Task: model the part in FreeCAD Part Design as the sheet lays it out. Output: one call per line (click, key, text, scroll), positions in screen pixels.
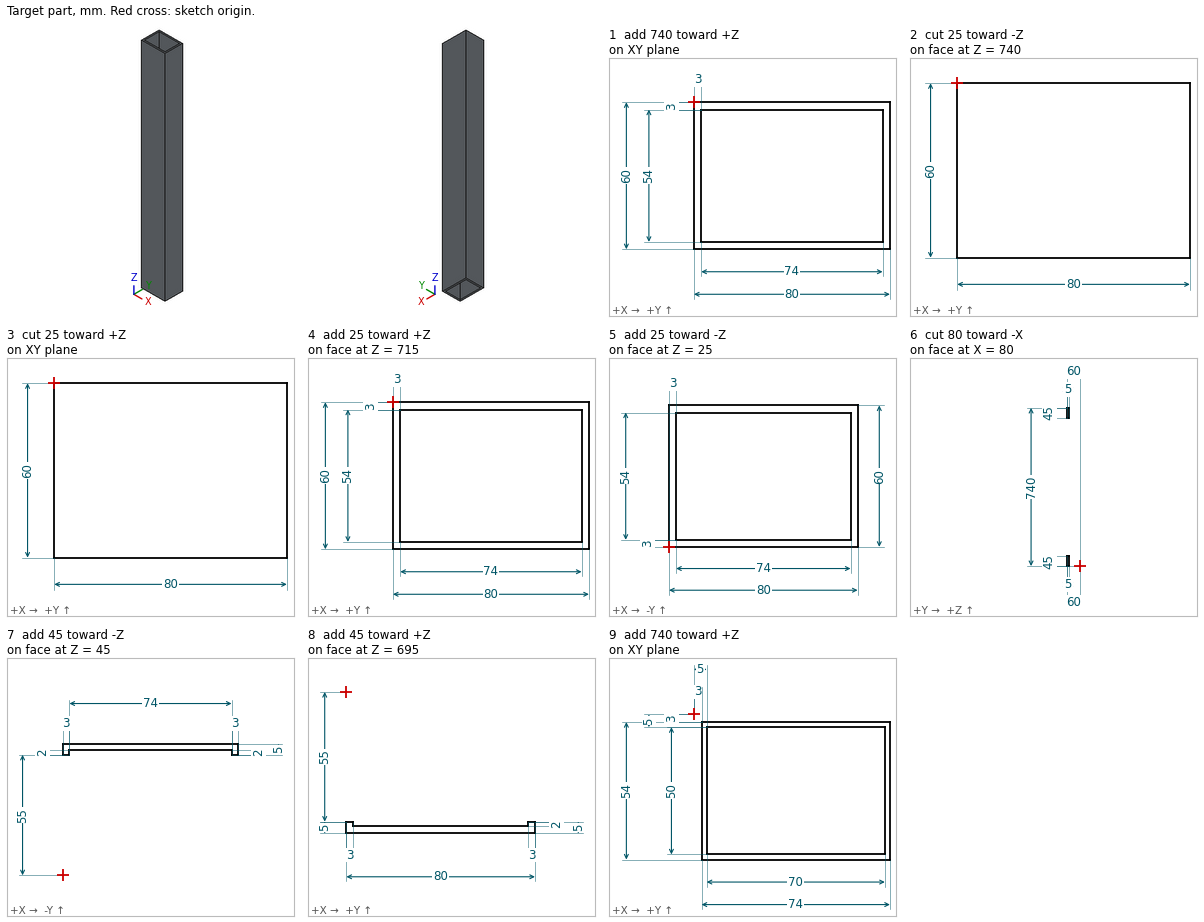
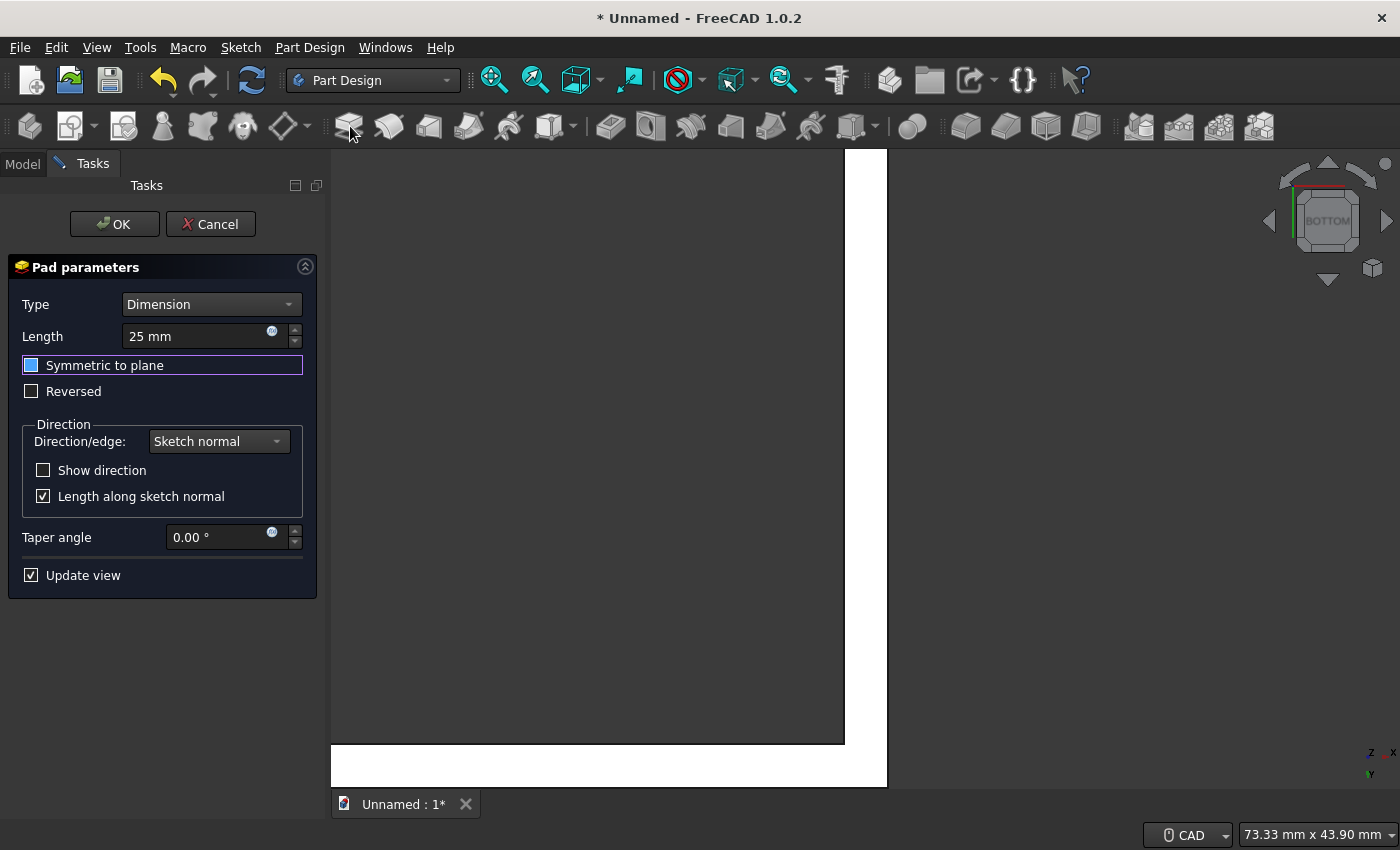
click(115, 224)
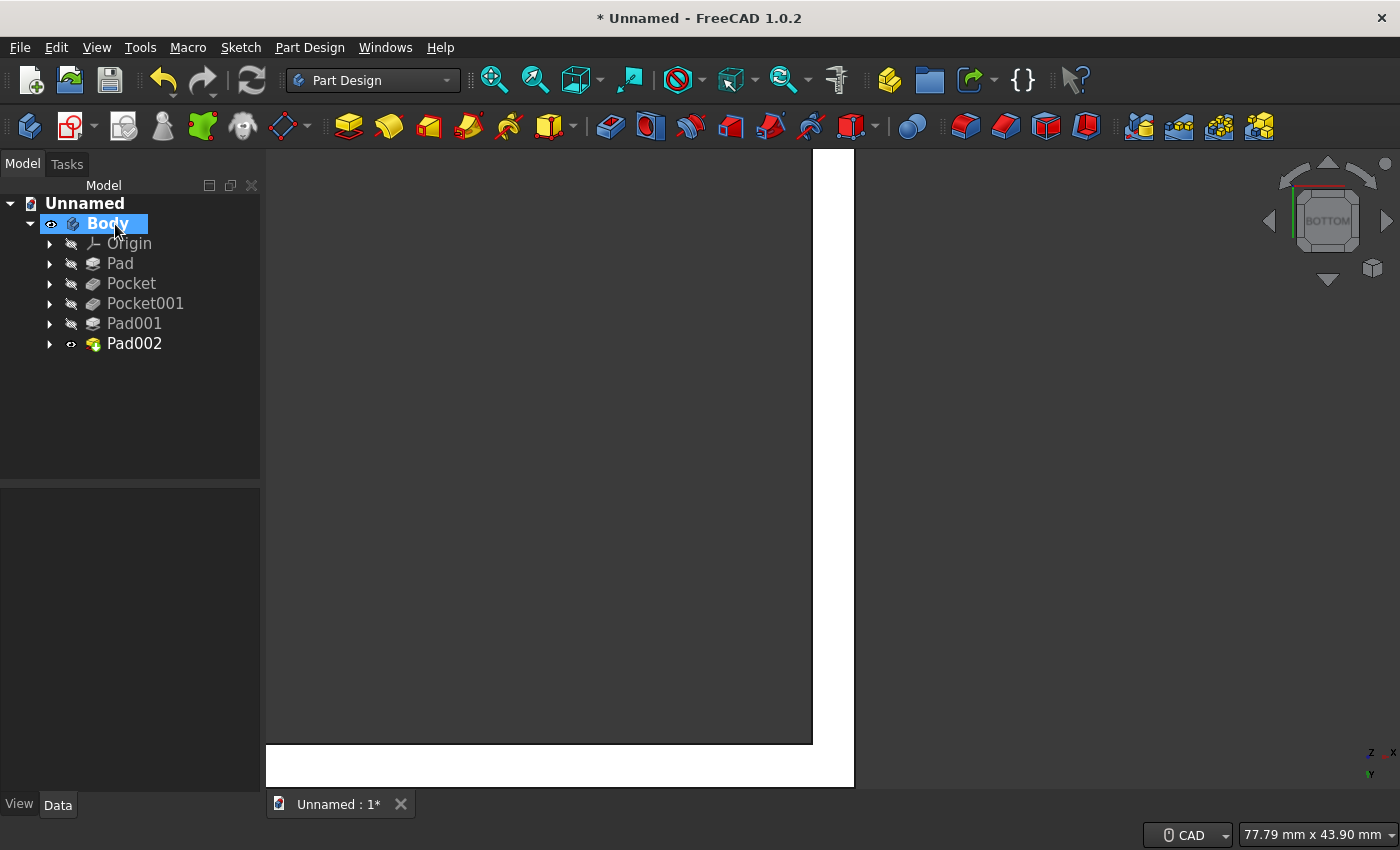
click(496, 80)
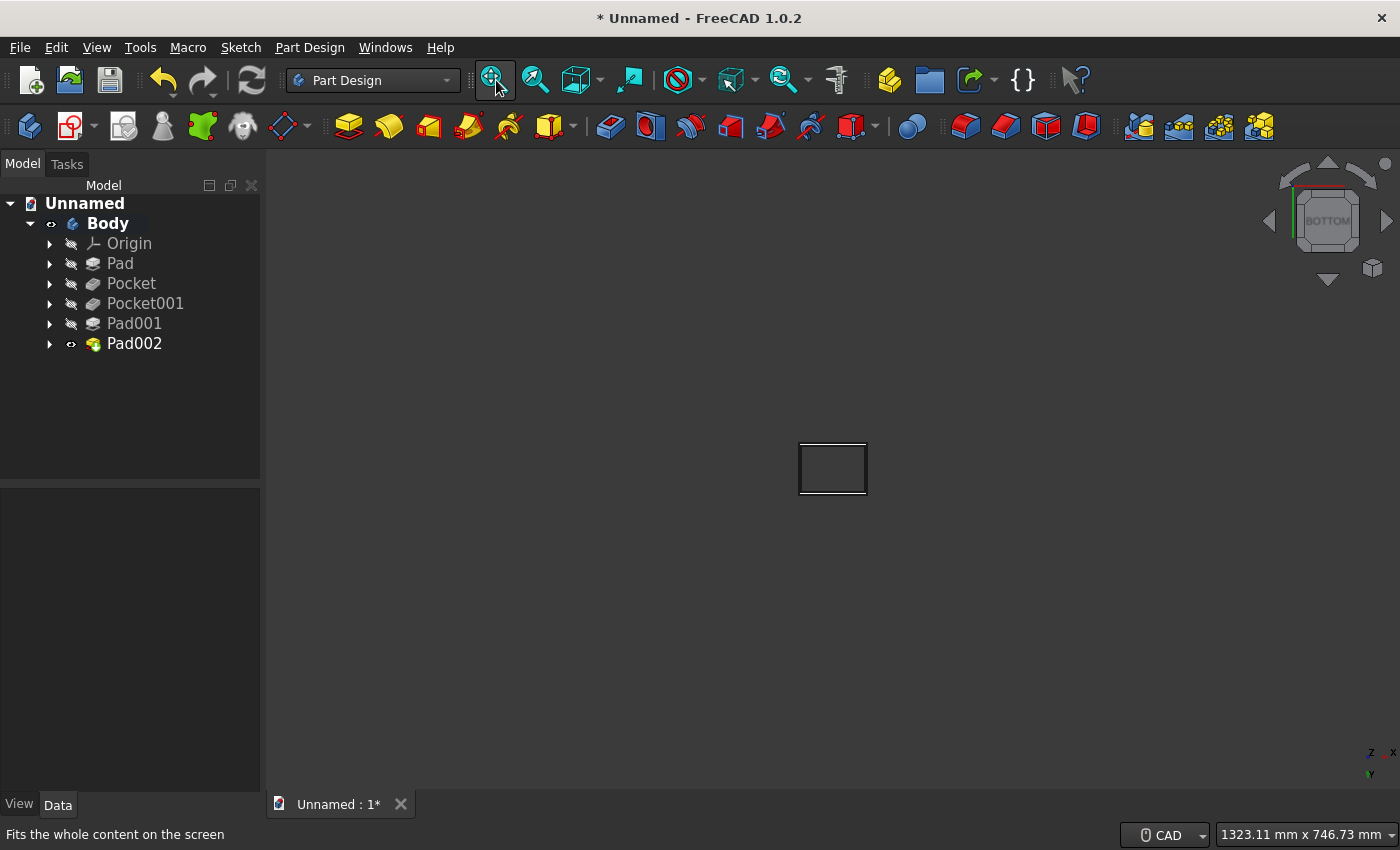
key(0)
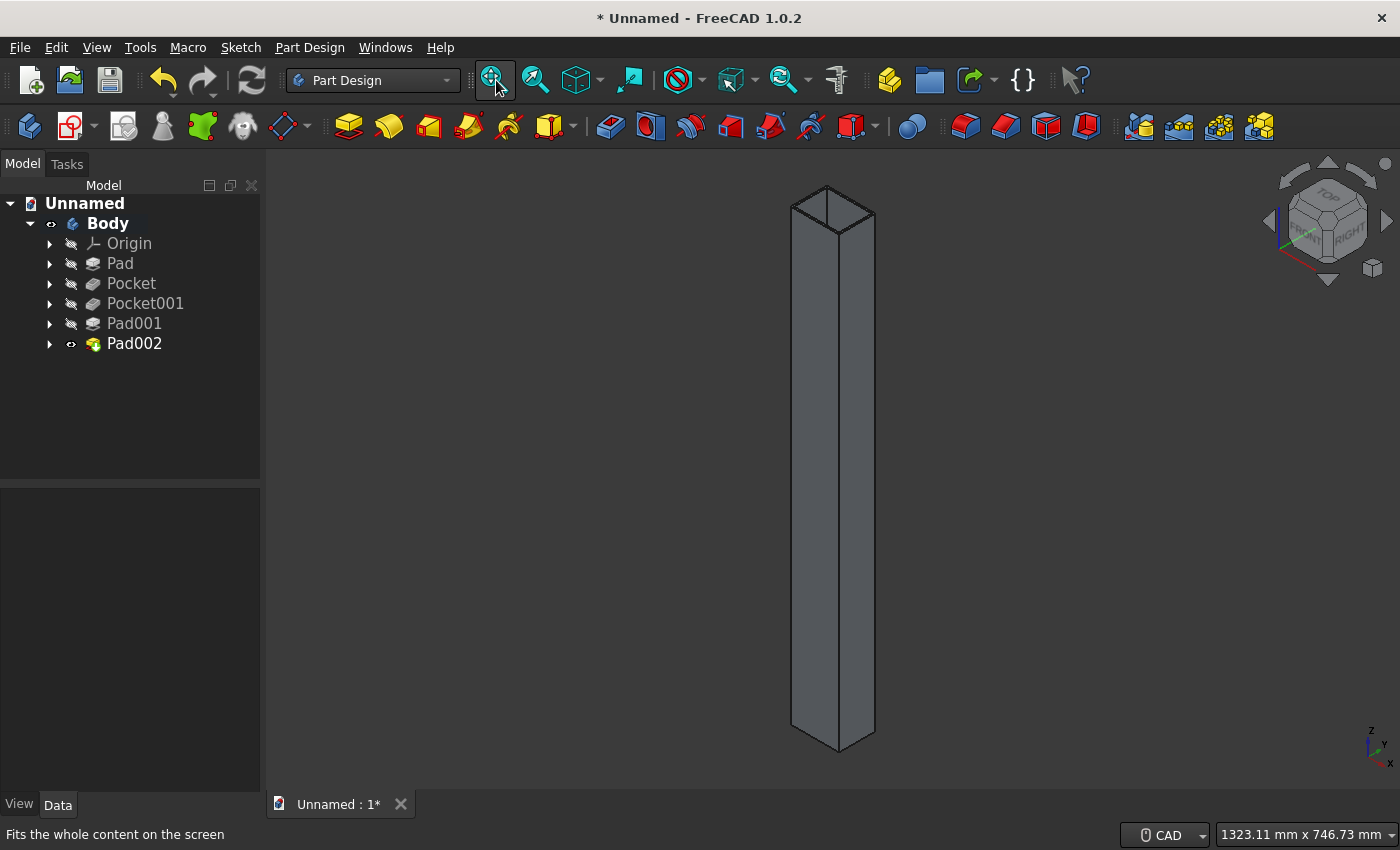
click(857, 260)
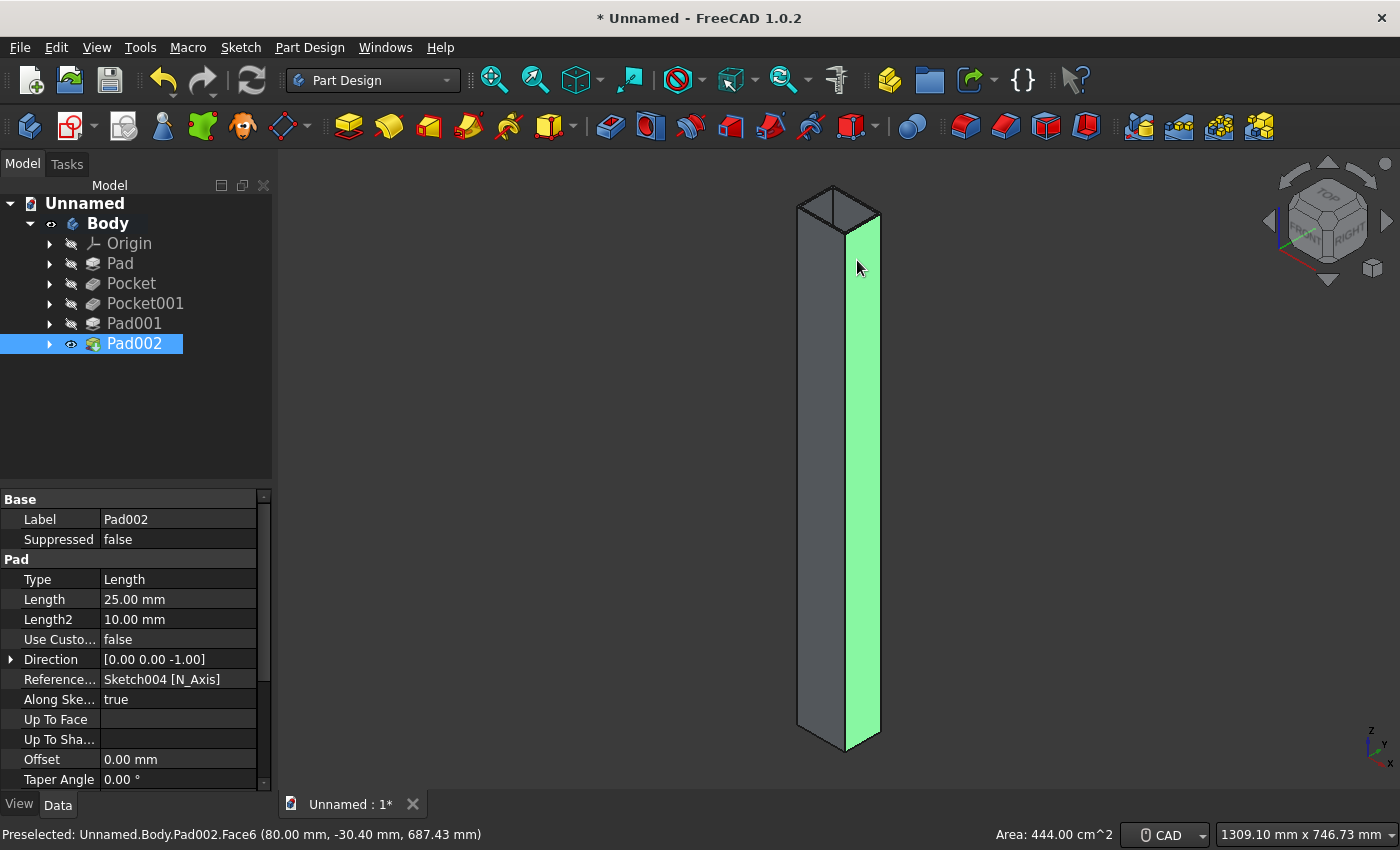
click(70, 126)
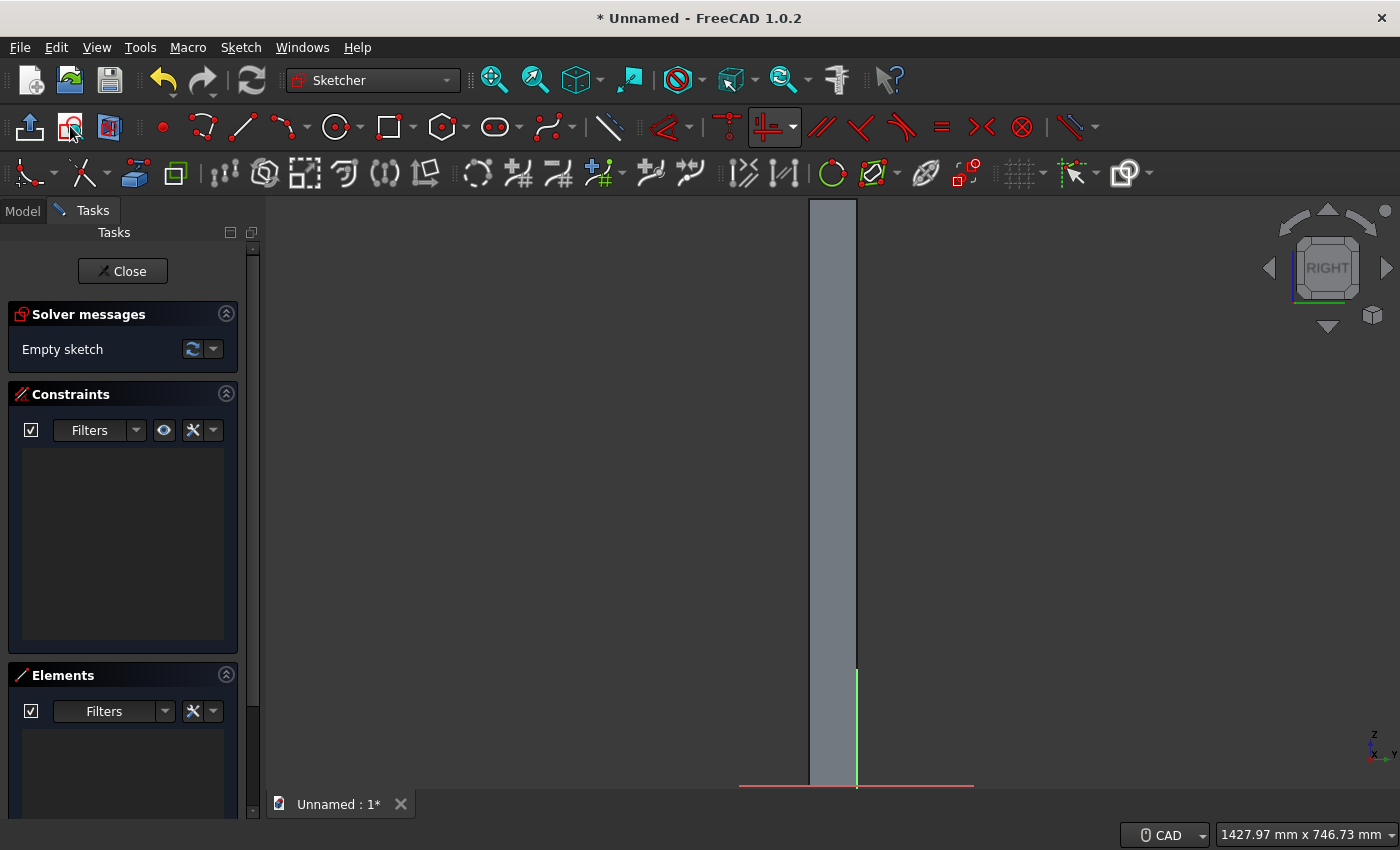
scroll(625, 493, down, 2)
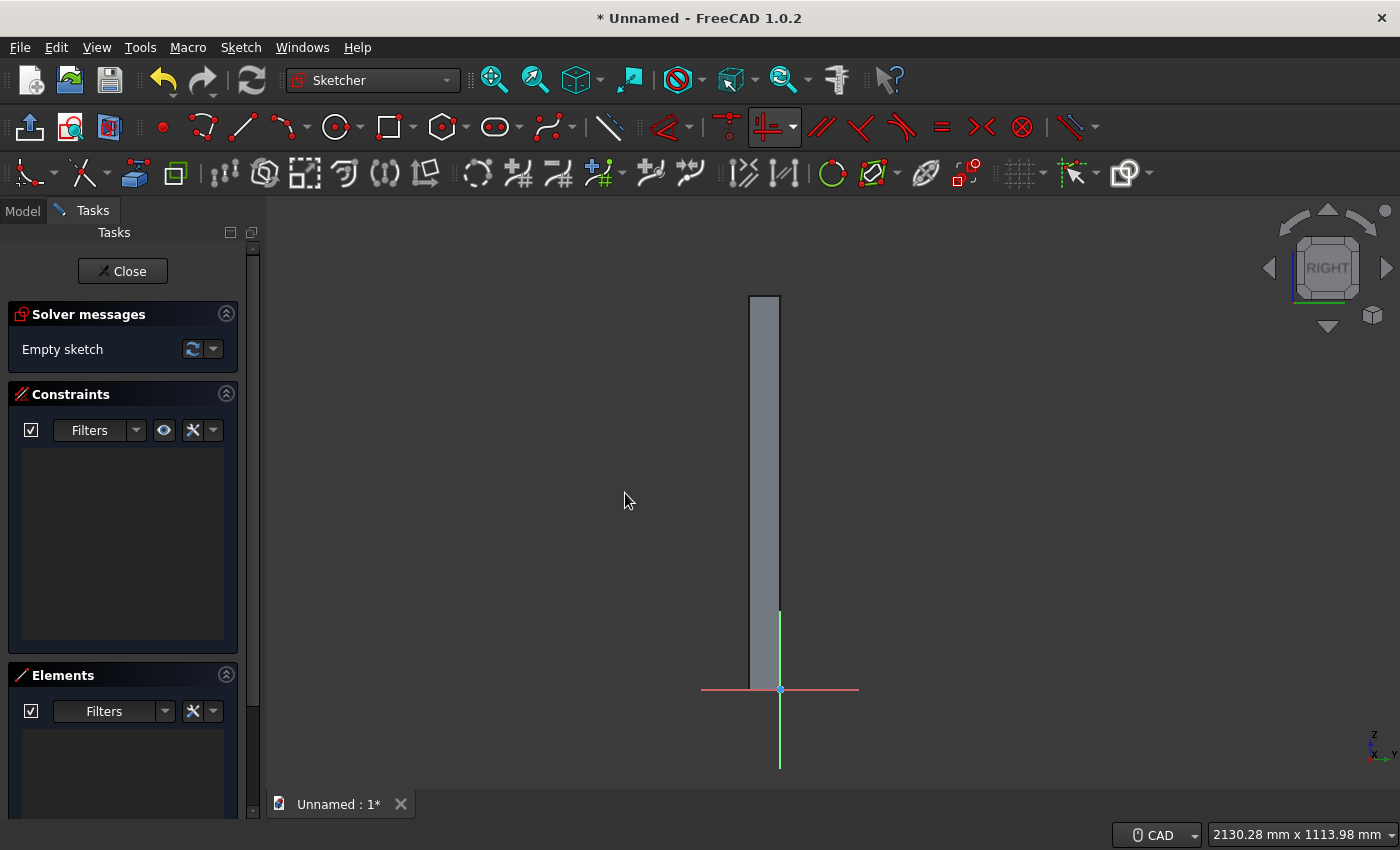
click(390, 128)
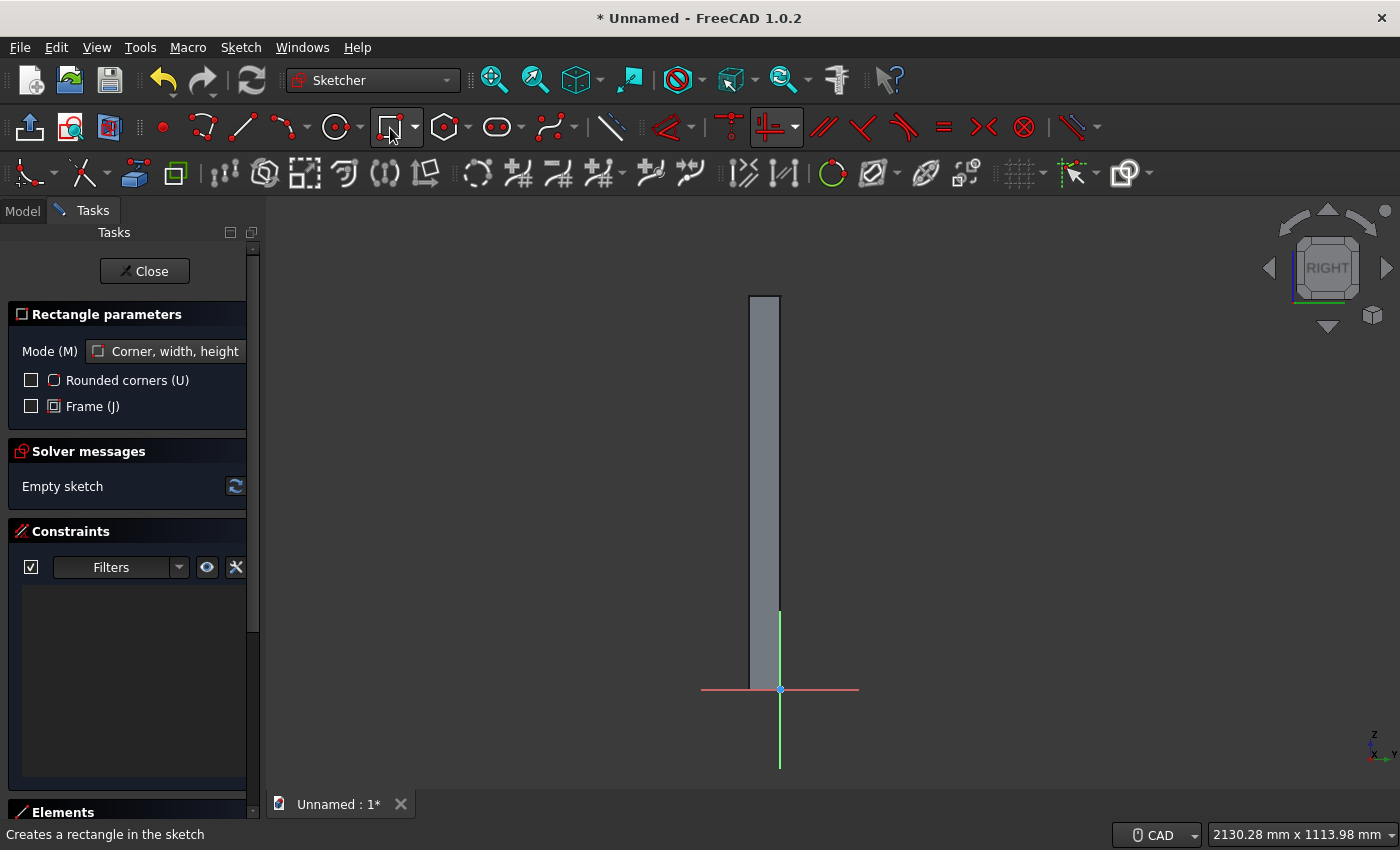
scroll(749, 296, up, 9)